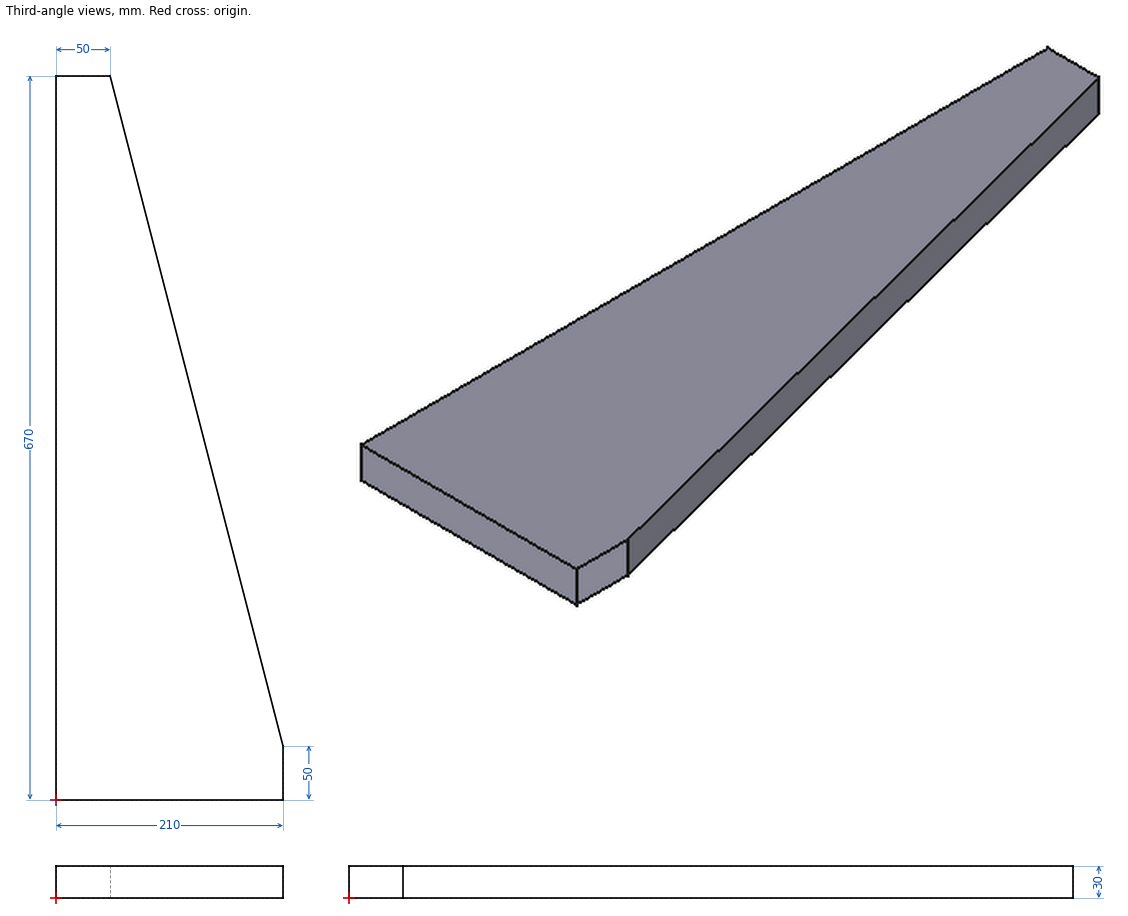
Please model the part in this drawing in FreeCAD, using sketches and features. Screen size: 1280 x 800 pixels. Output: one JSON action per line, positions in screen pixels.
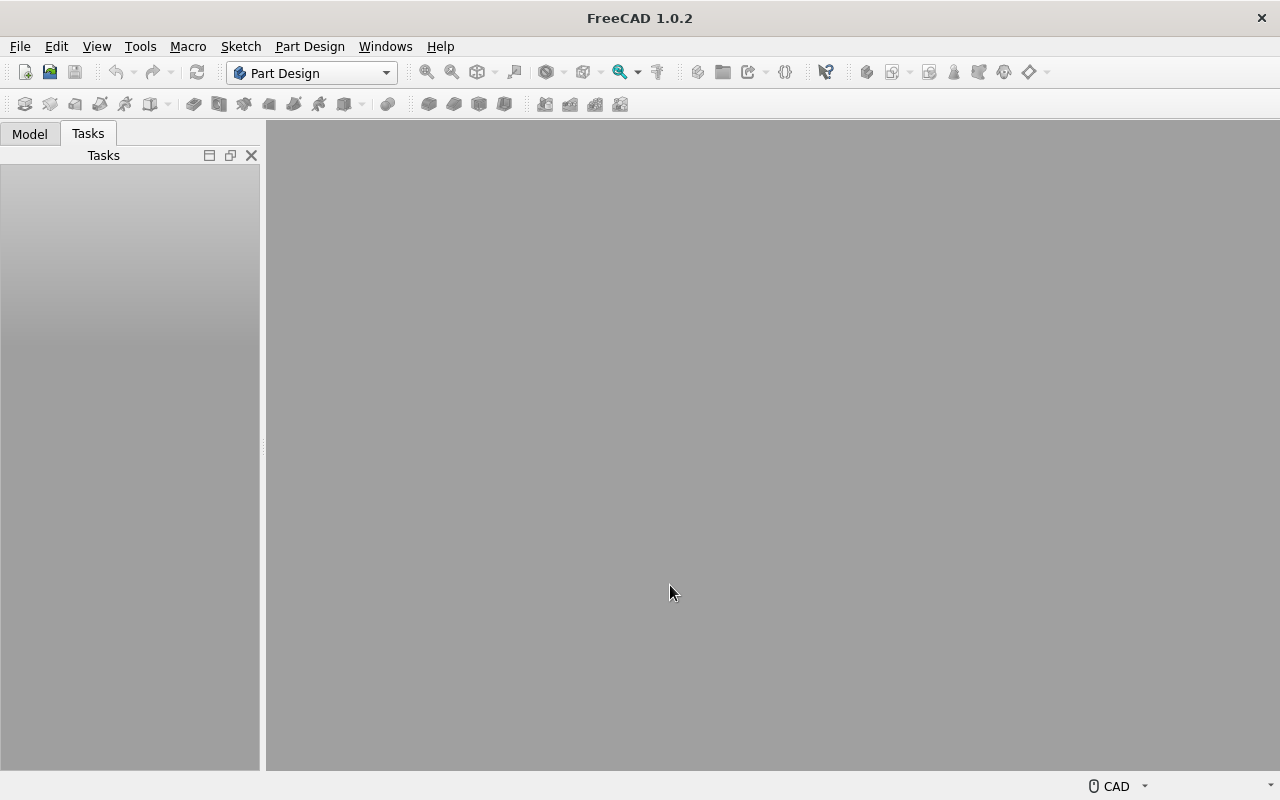
{"action": "key", "text": "ctrl+n"}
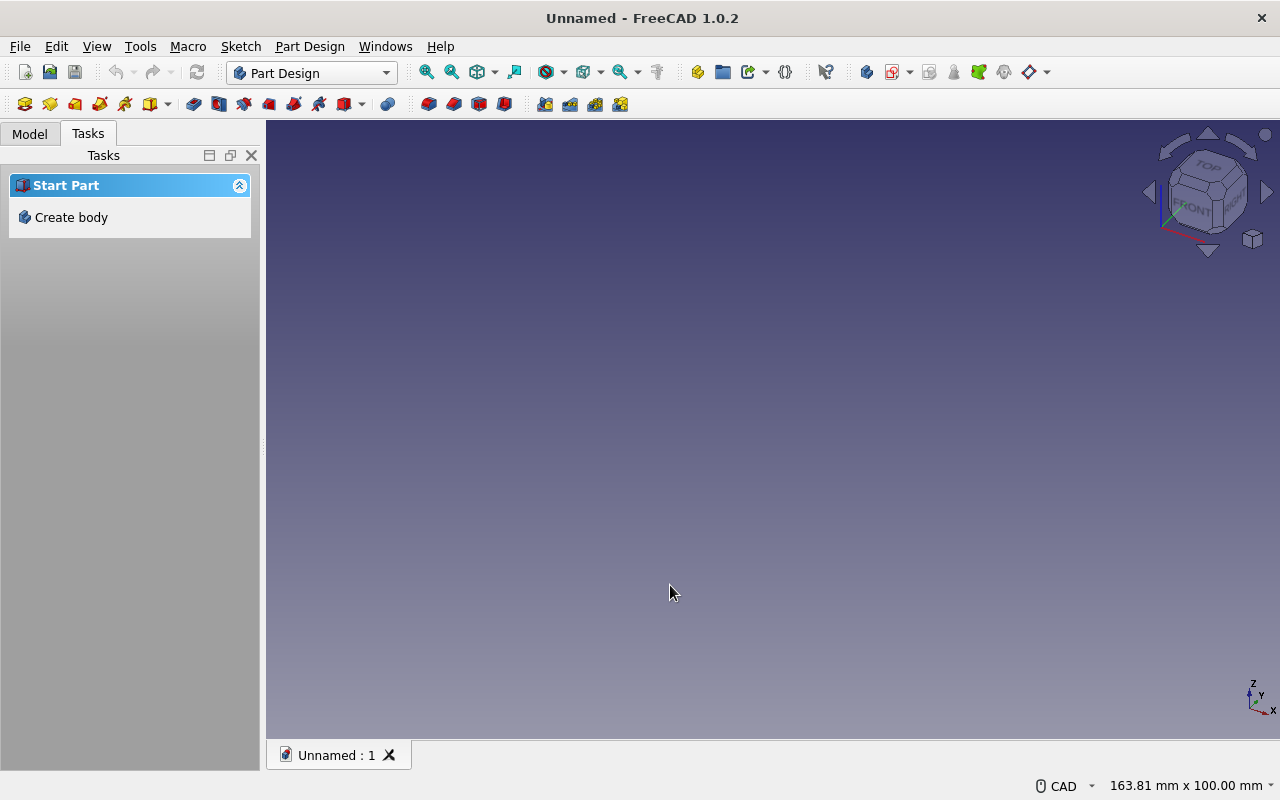
{"action": "left_click", "coordinate": [892, 72]}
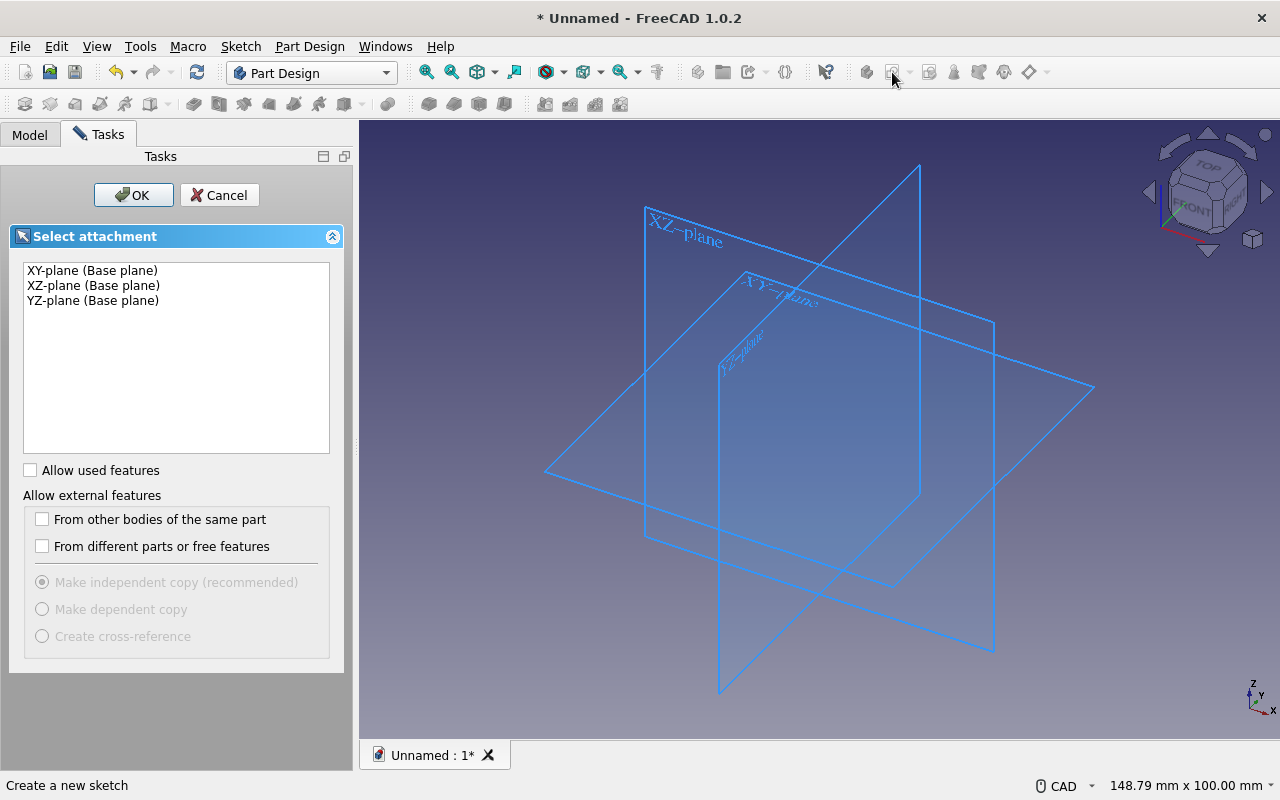
{"action": "left_click", "coordinate": [84, 270]}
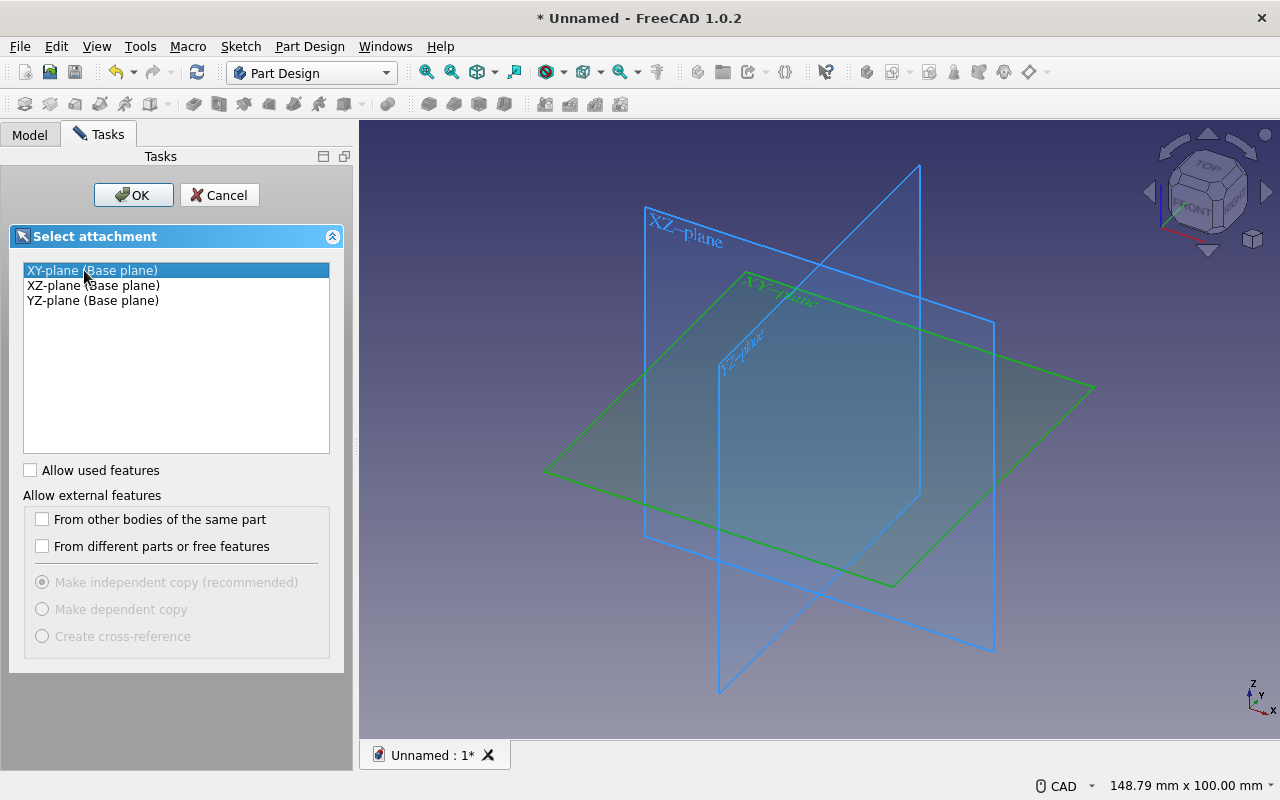
{"action": "left_click", "coordinate": [134, 195]}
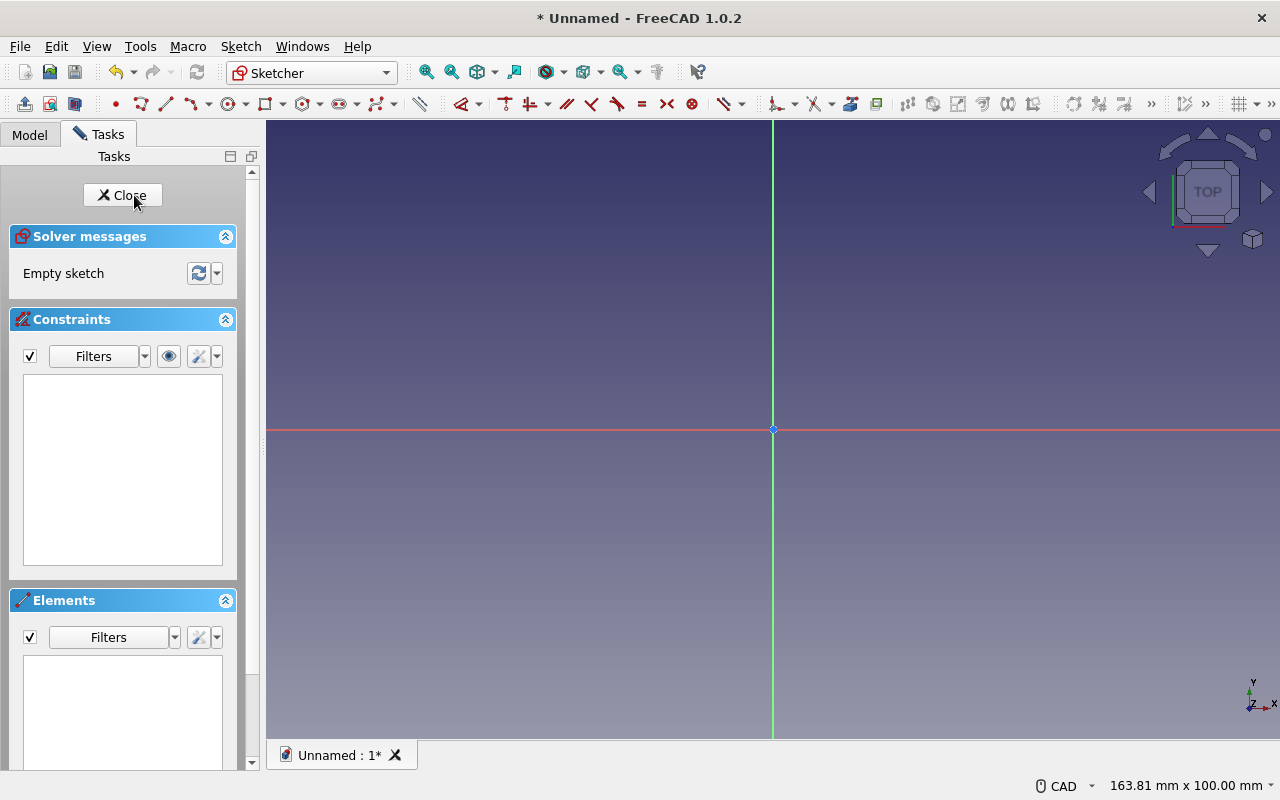
{"action": "scroll", "coordinate": [633, 636], "scroll_direction": "down", "scroll_amount": 12}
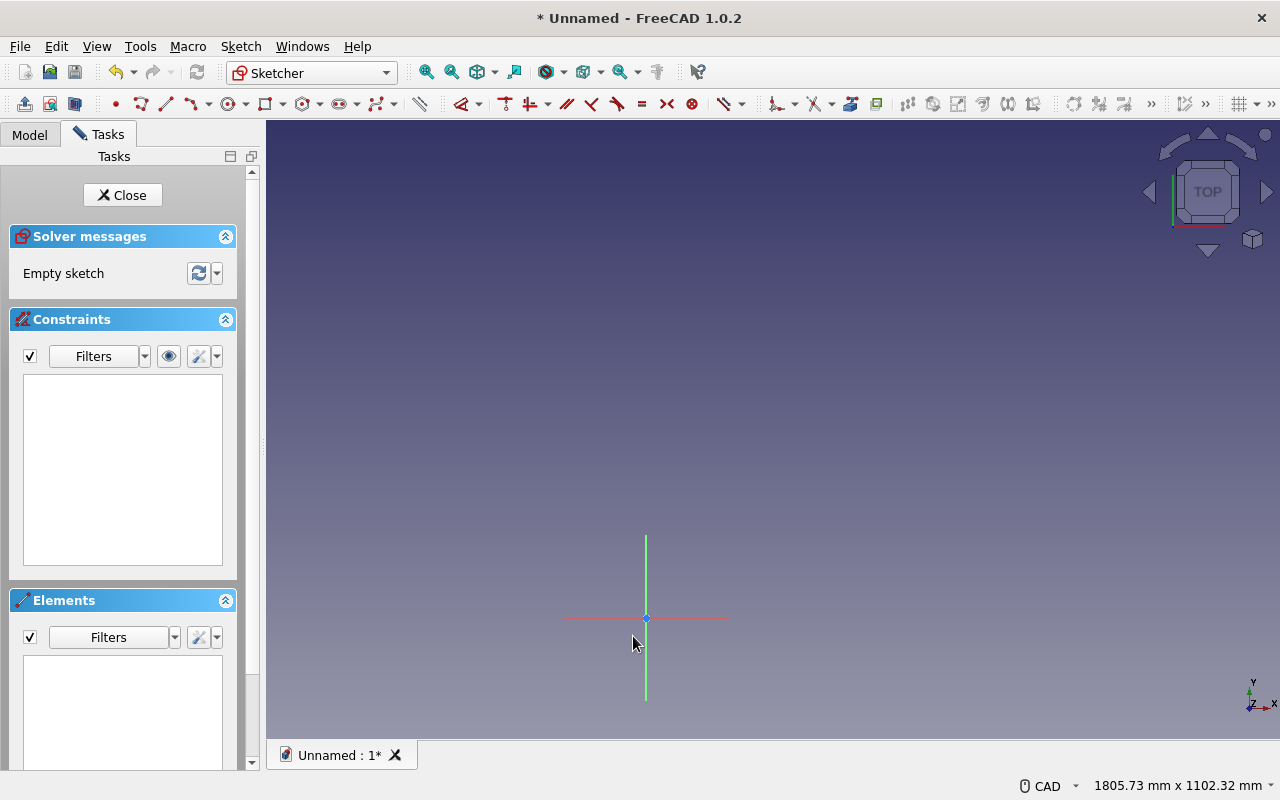
{"action": "left_click", "coordinate": [141, 104]}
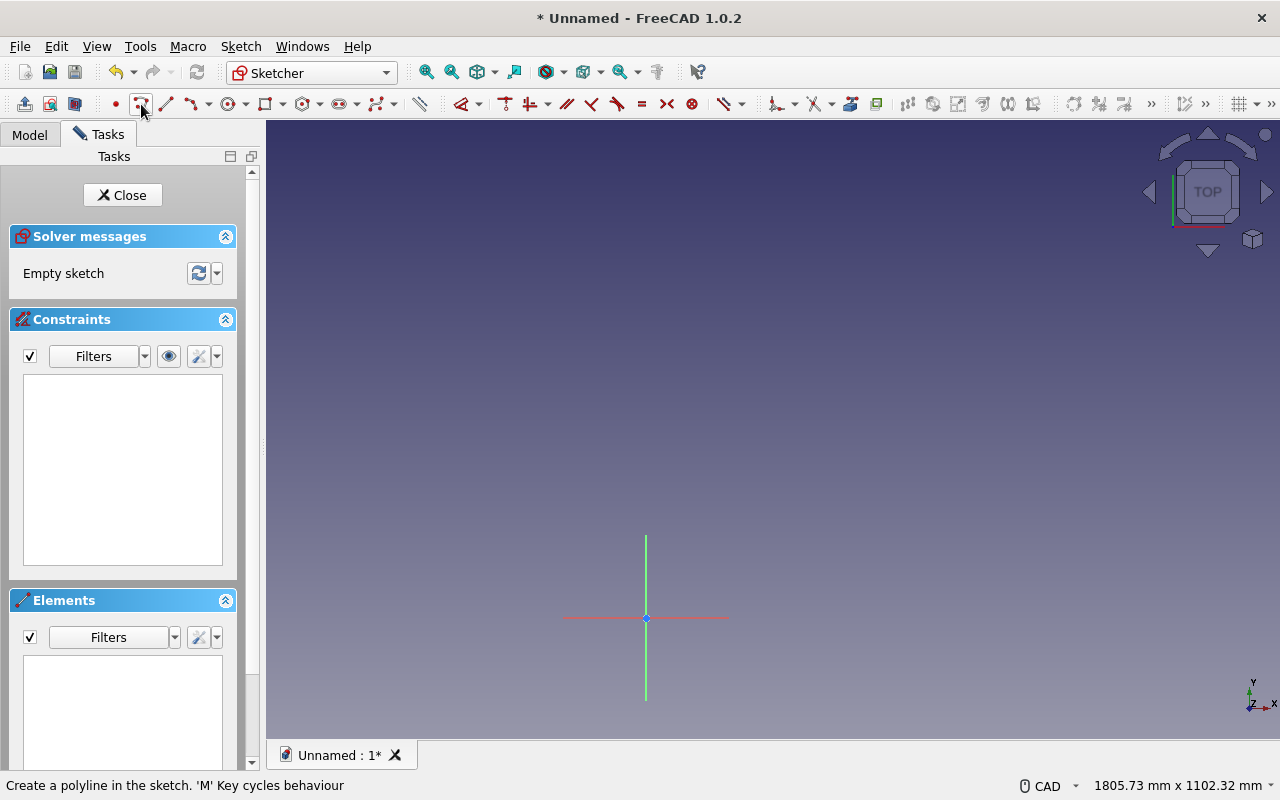
{"action": "left_click", "coordinate": [646, 618]}
{"action": "left_click", "coordinate": [764, 609]}
{"action": "left_click", "coordinate": [764, 590]}
{"action": "left_click", "coordinate": [674, 242]}
{"action": "left_click", "coordinate": [655, 242]}
{"action": "left_click", "coordinate": [646, 618]}
{"action": "key", "text": "Escape"}
{"action": "key", "text": "Escape"}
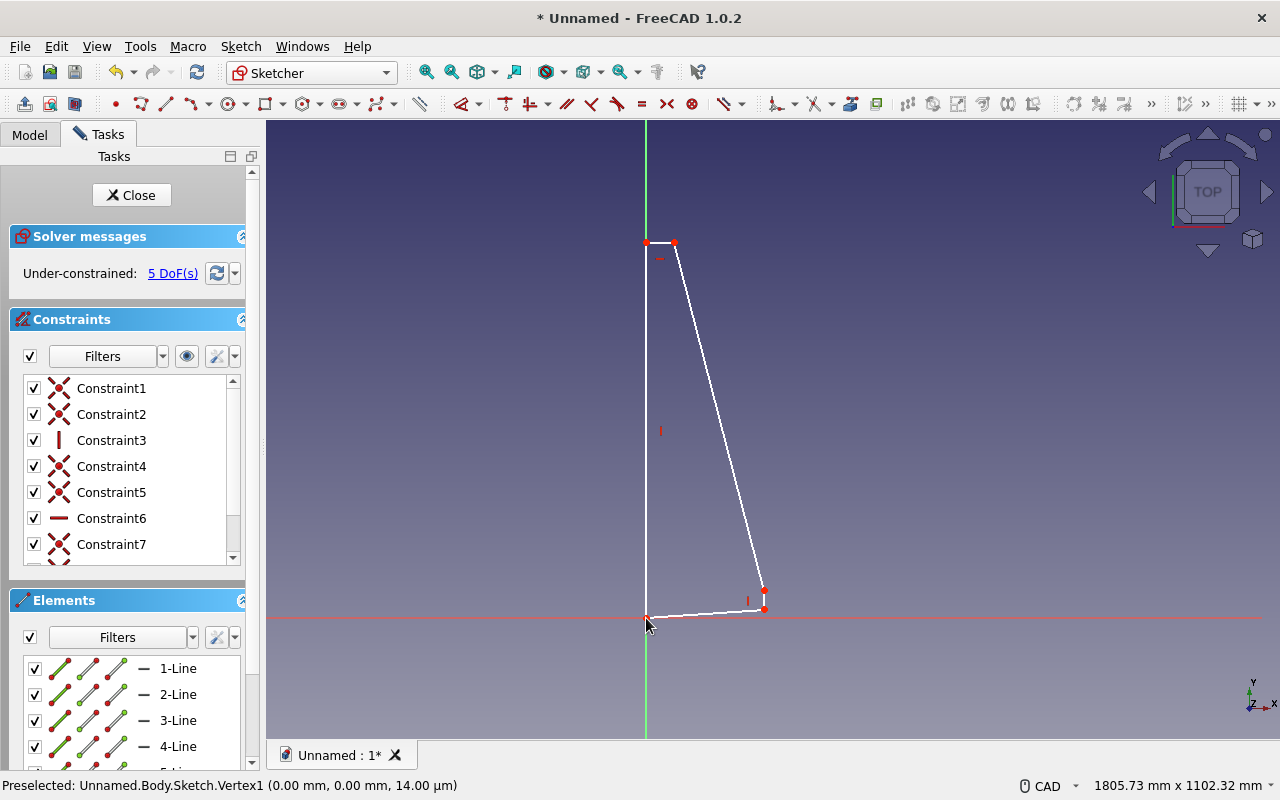
{"action": "left_click", "coordinate": [681, 616]}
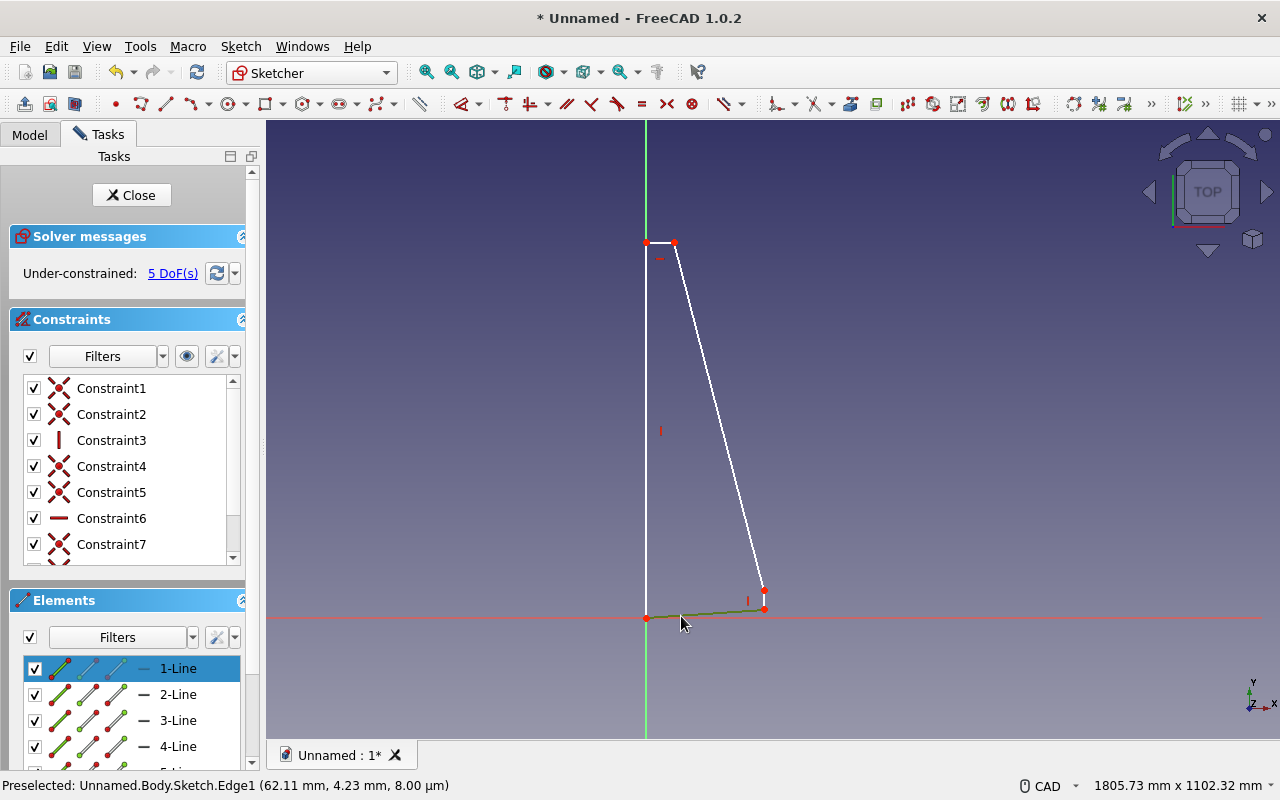
{"action": "left_click", "coordinate": [548, 104]}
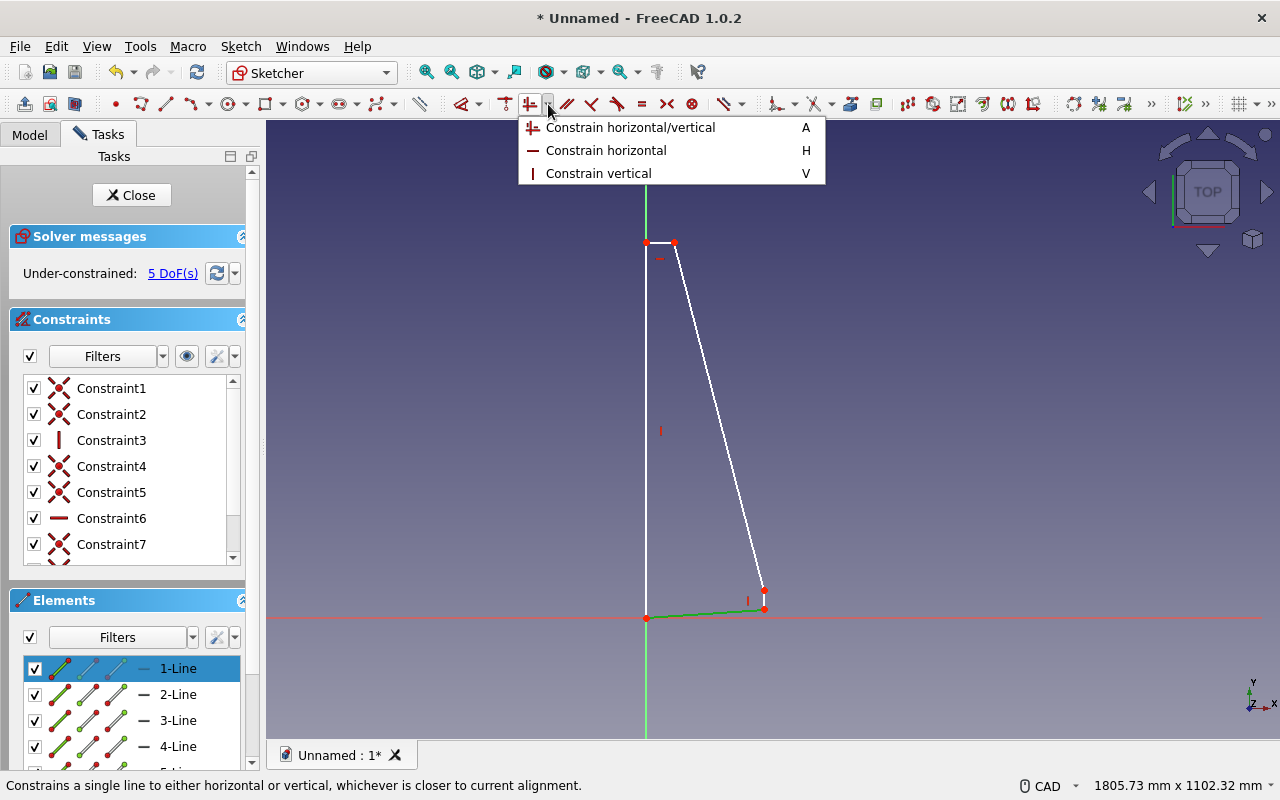
{"action": "left_click", "coordinate": [672, 150]}